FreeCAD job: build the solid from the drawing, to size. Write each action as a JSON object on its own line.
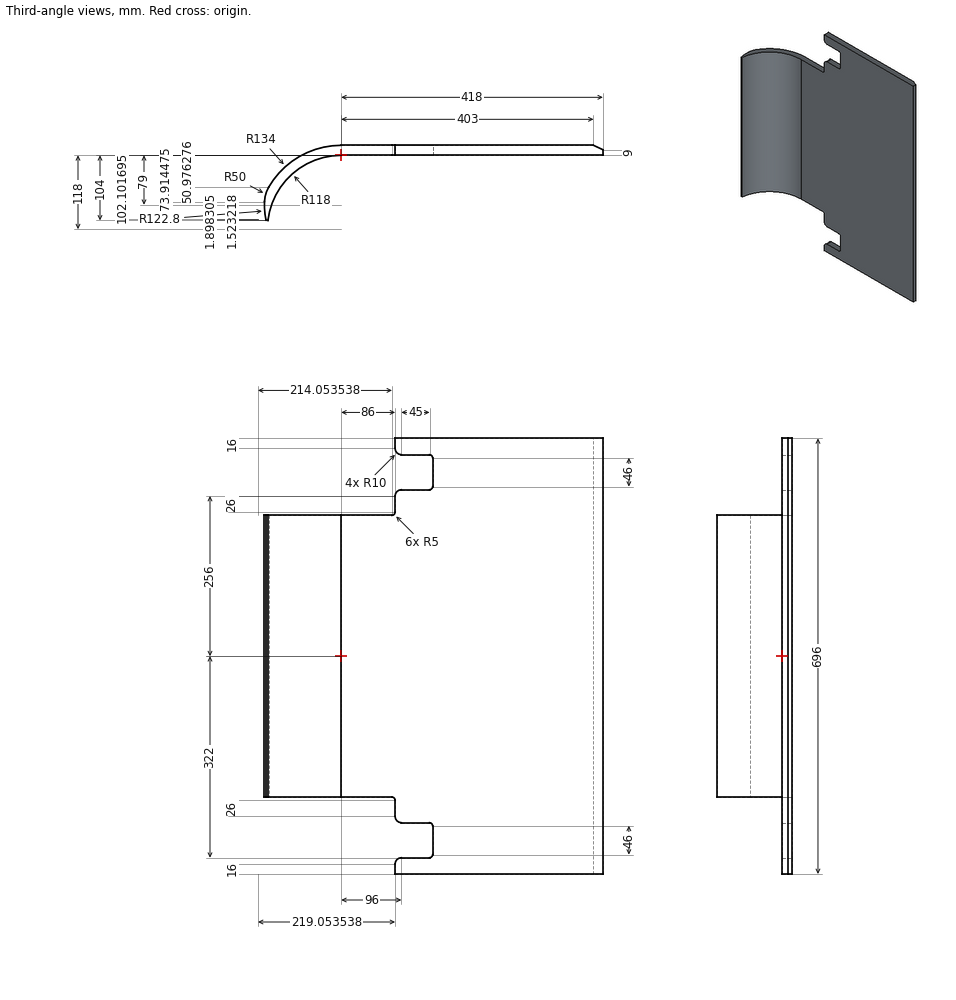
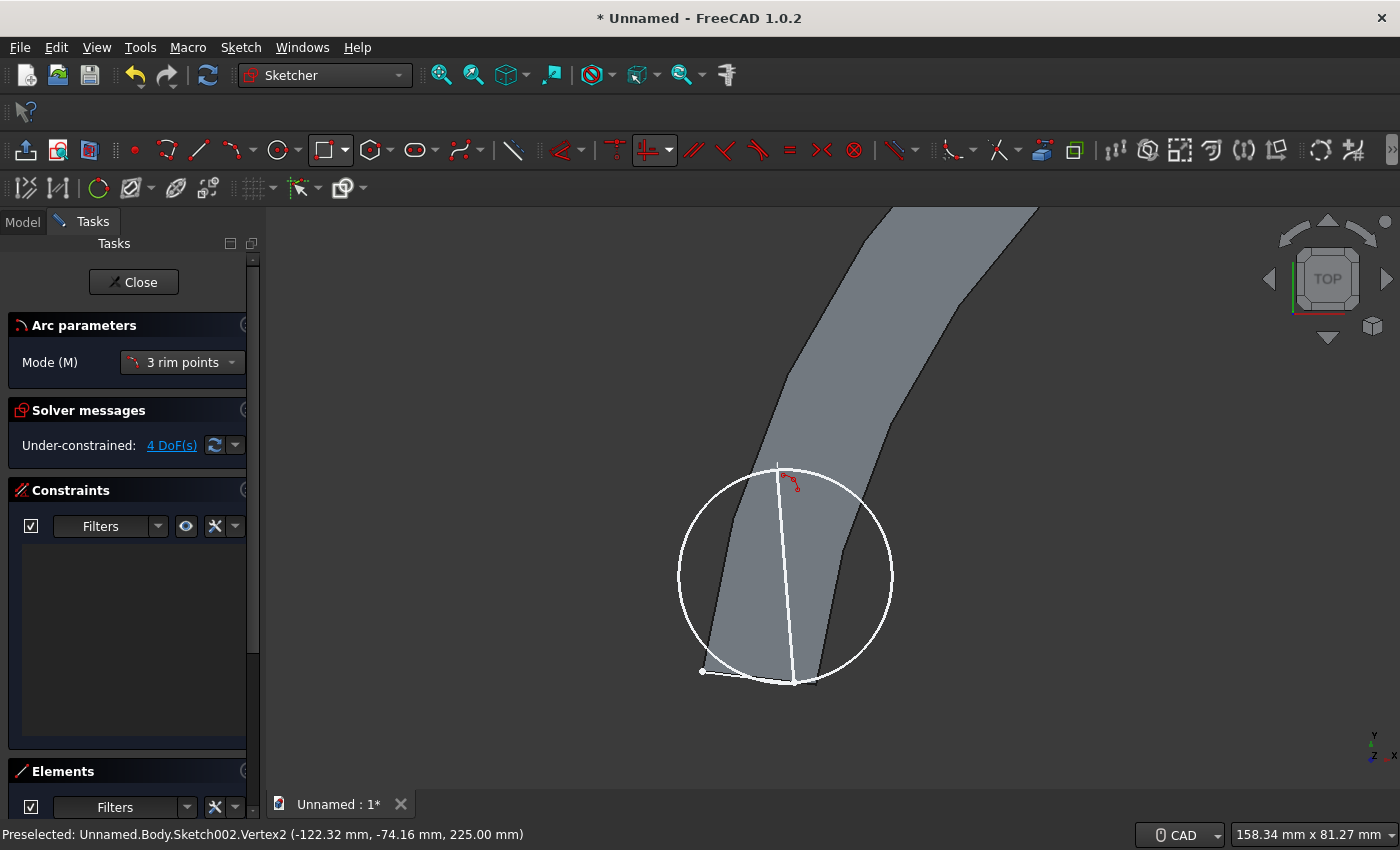
{"action": "scroll", "coordinate": [779, 576], "scroll_direction": "up", "scroll_amount": 5}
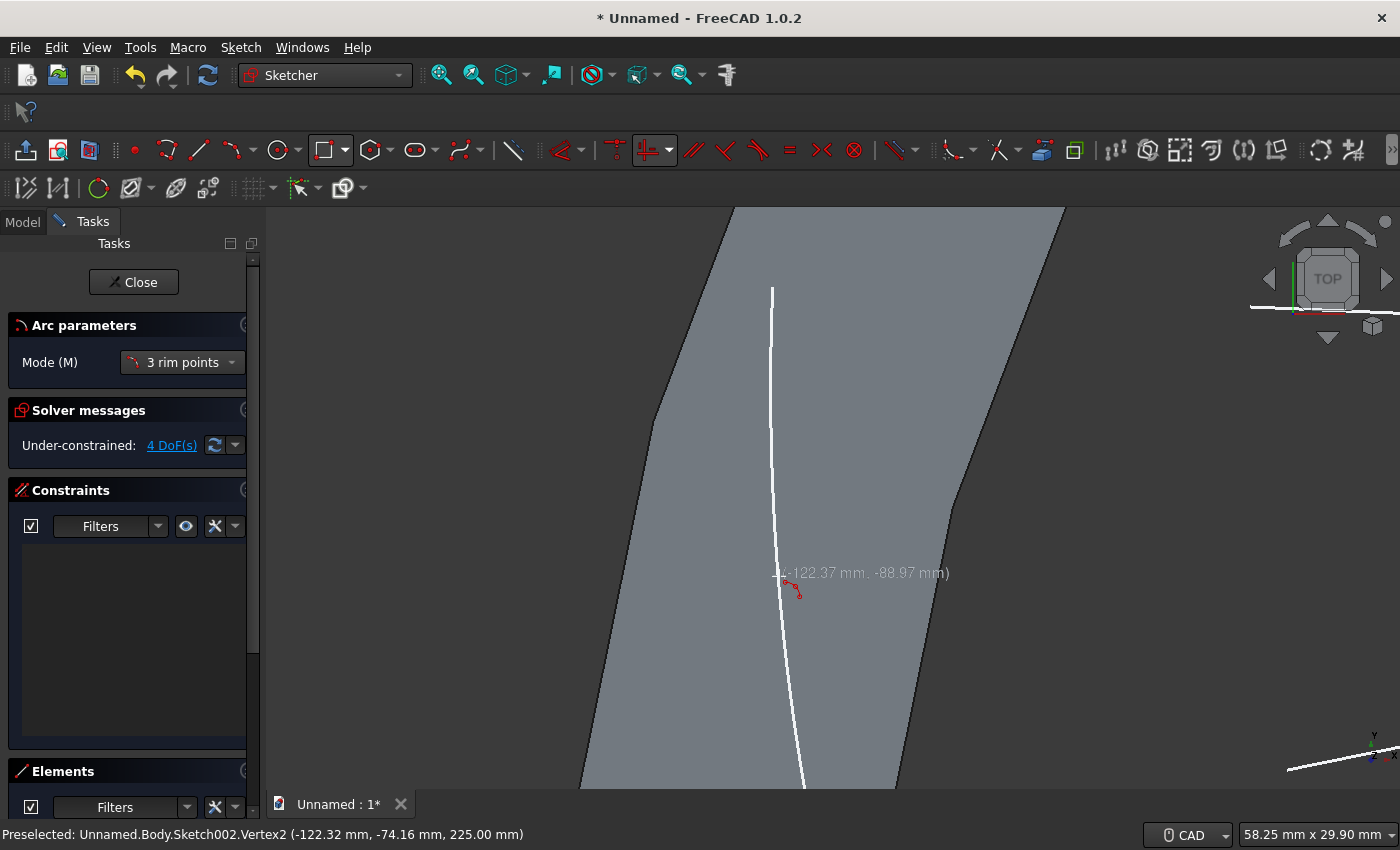
{"action": "left_click", "coordinate": [777, 575]}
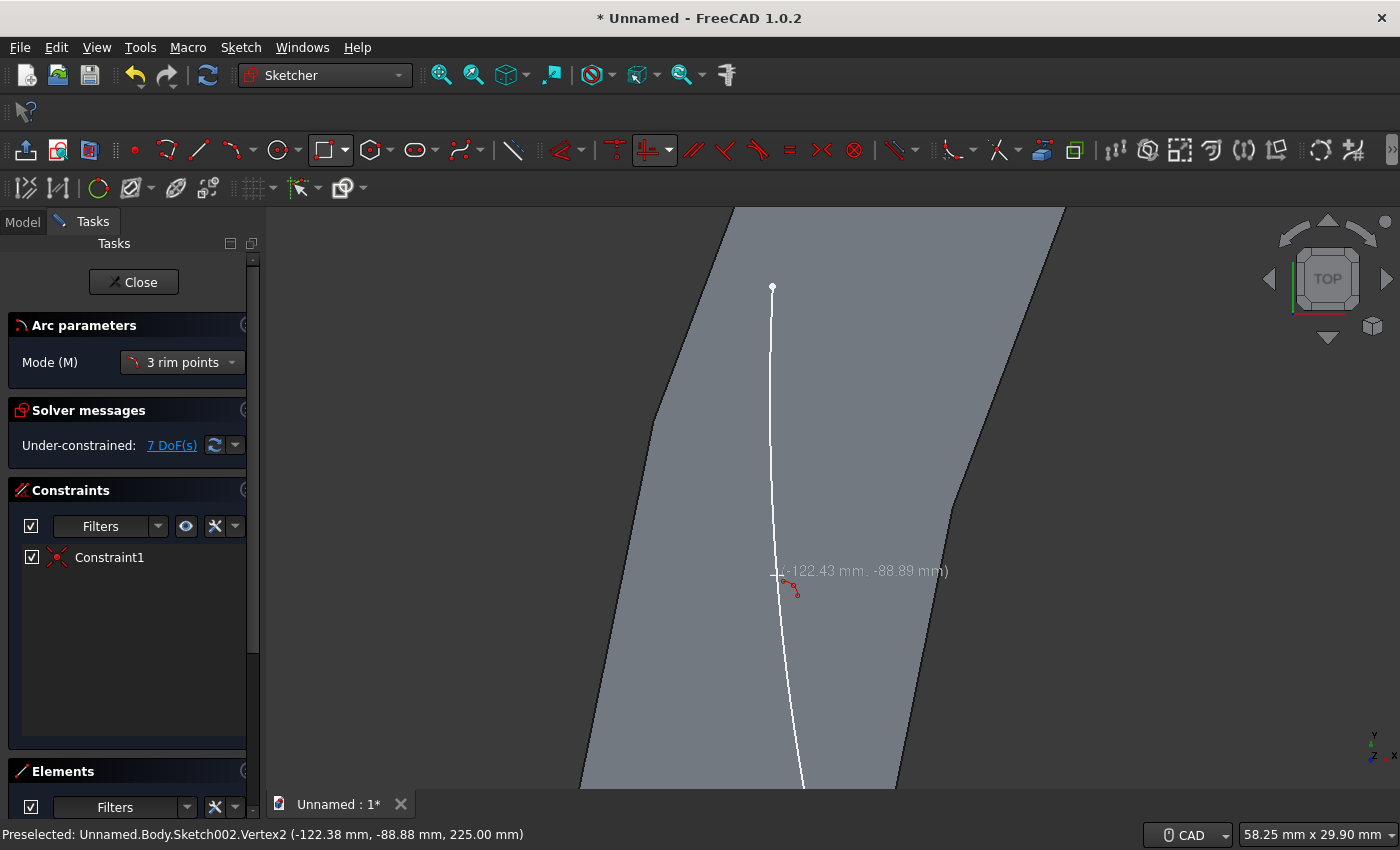
{"action": "left_click", "coordinate": [773, 287]}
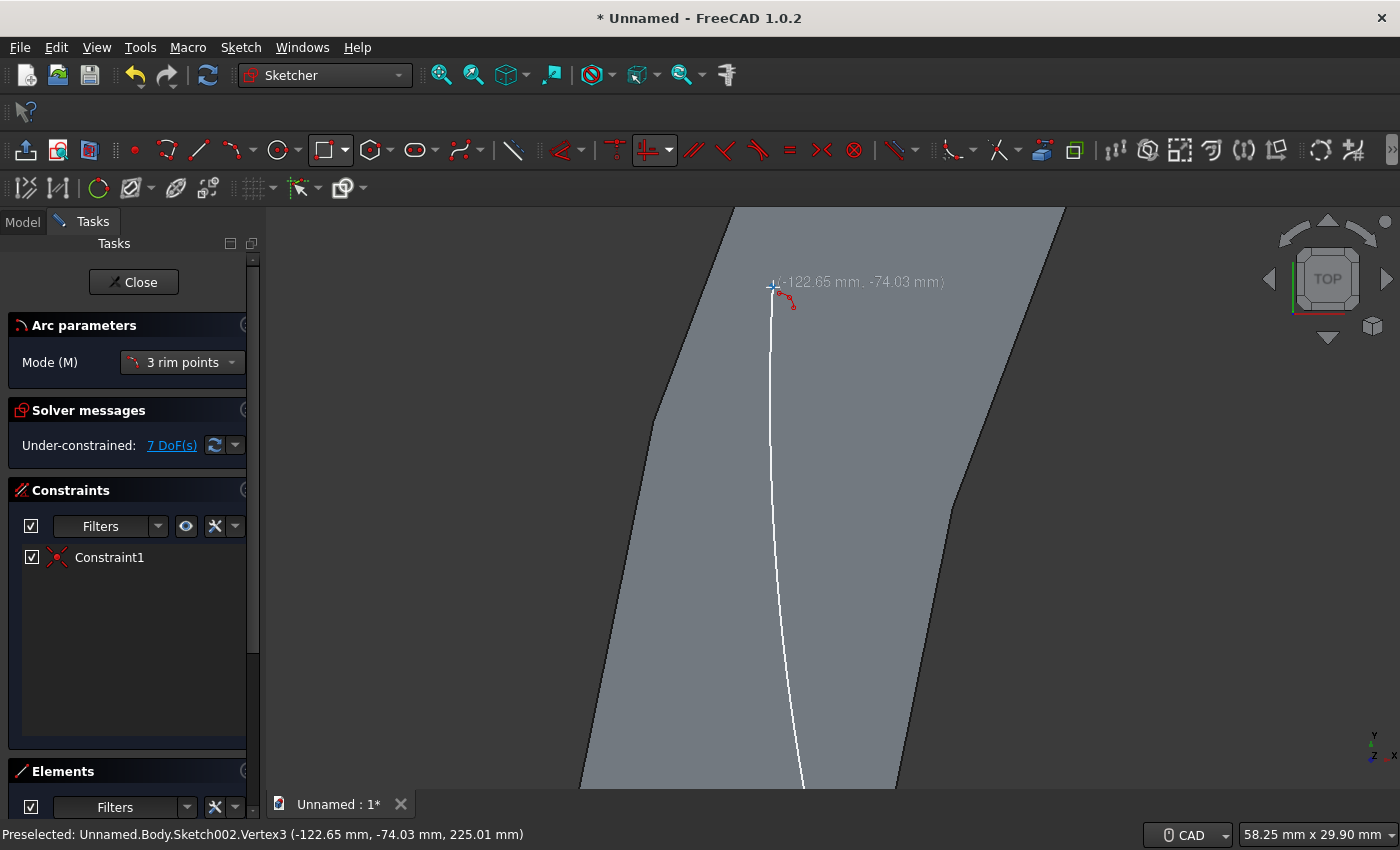
{"action": "scroll", "coordinate": [781, 584], "scroll_direction": "down", "scroll_amount": 5}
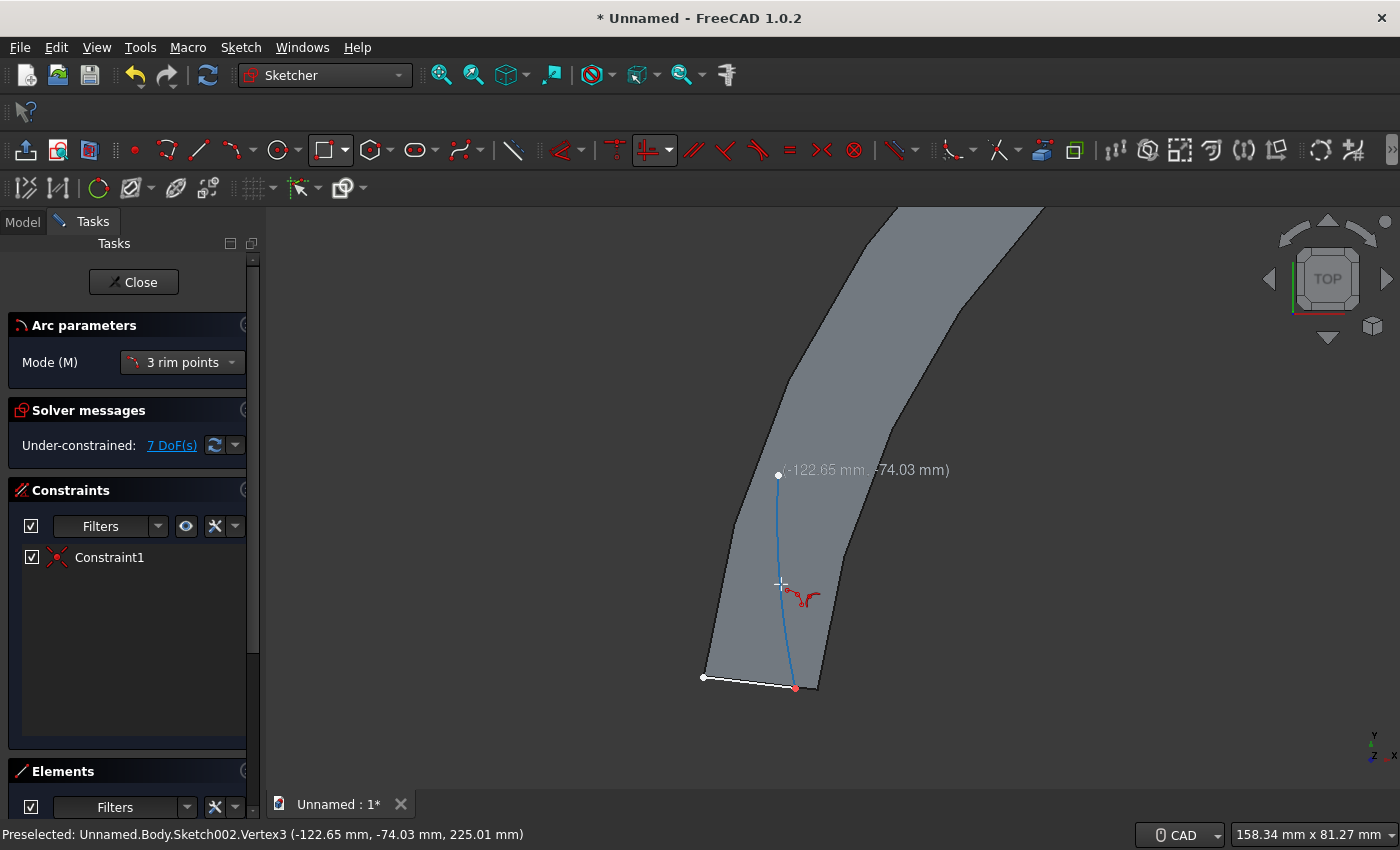
{"action": "left_click", "coordinate": [826, 310]}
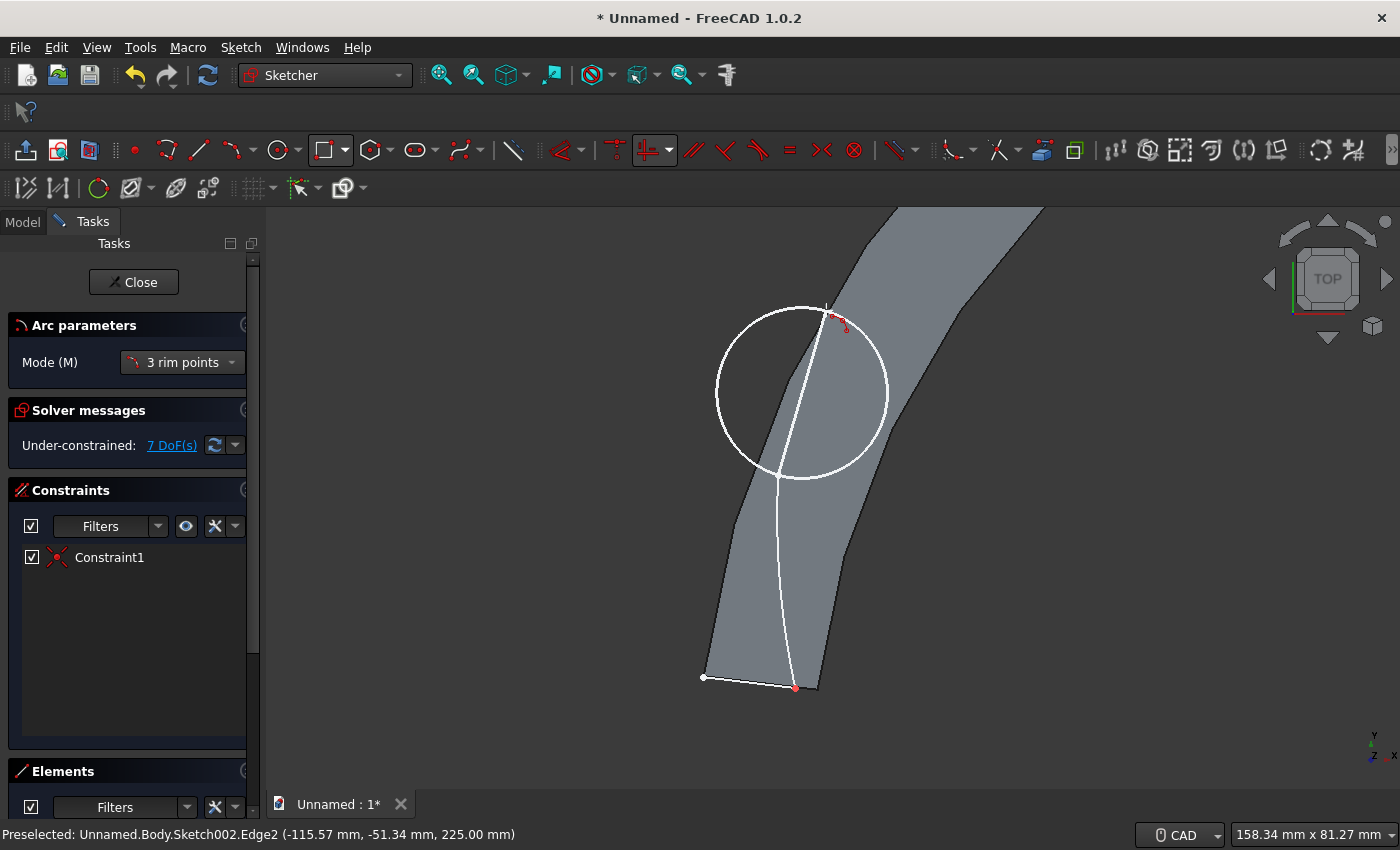
{"action": "scroll", "coordinate": [792, 389], "scroll_direction": "up", "scroll_amount": 3}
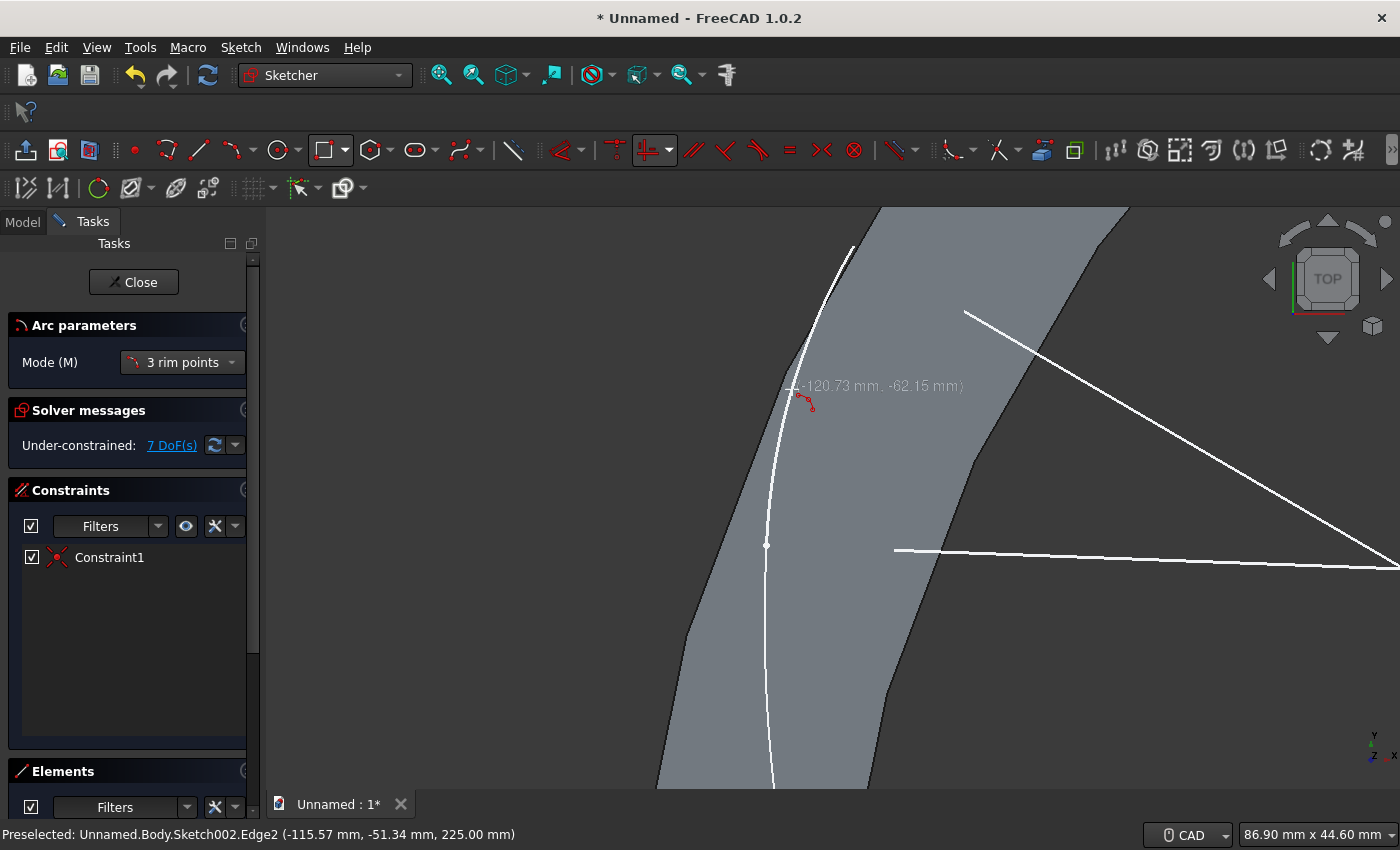
{"action": "left_click", "coordinate": [791, 389]}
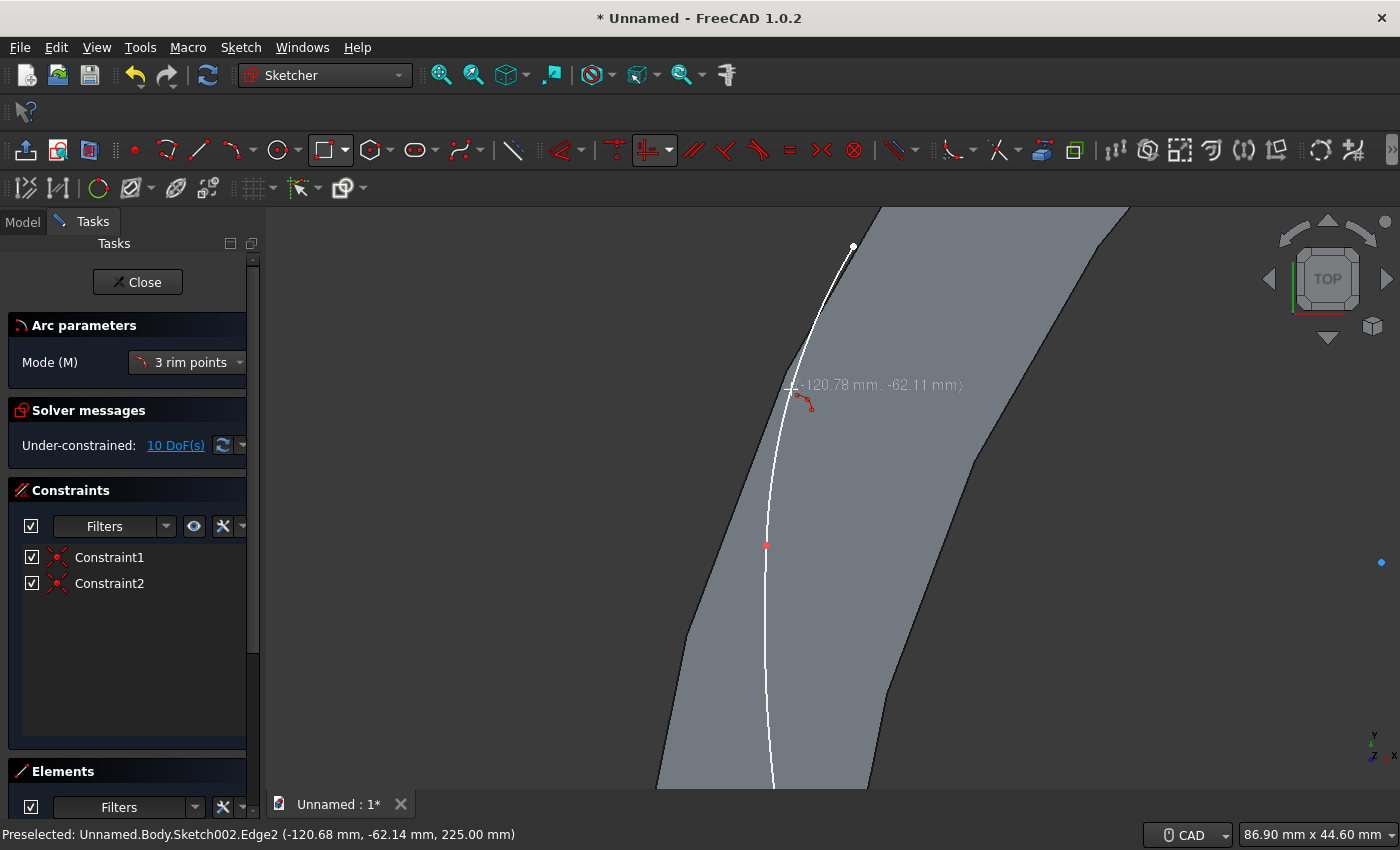
{"action": "left_click", "coordinate": [854, 247]}